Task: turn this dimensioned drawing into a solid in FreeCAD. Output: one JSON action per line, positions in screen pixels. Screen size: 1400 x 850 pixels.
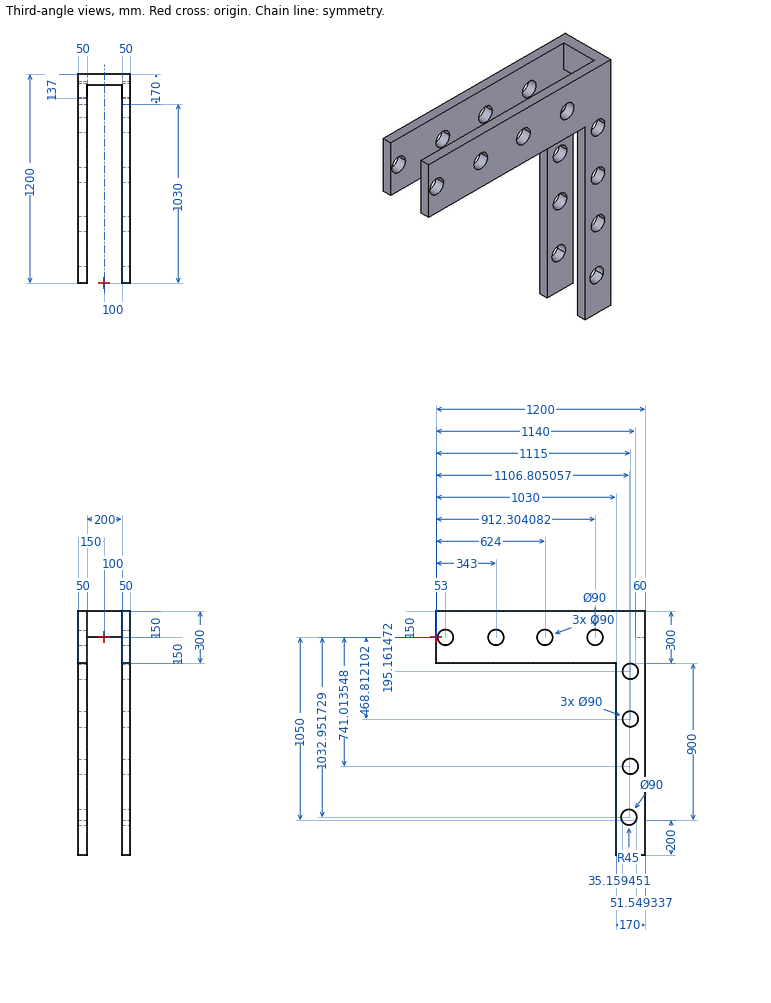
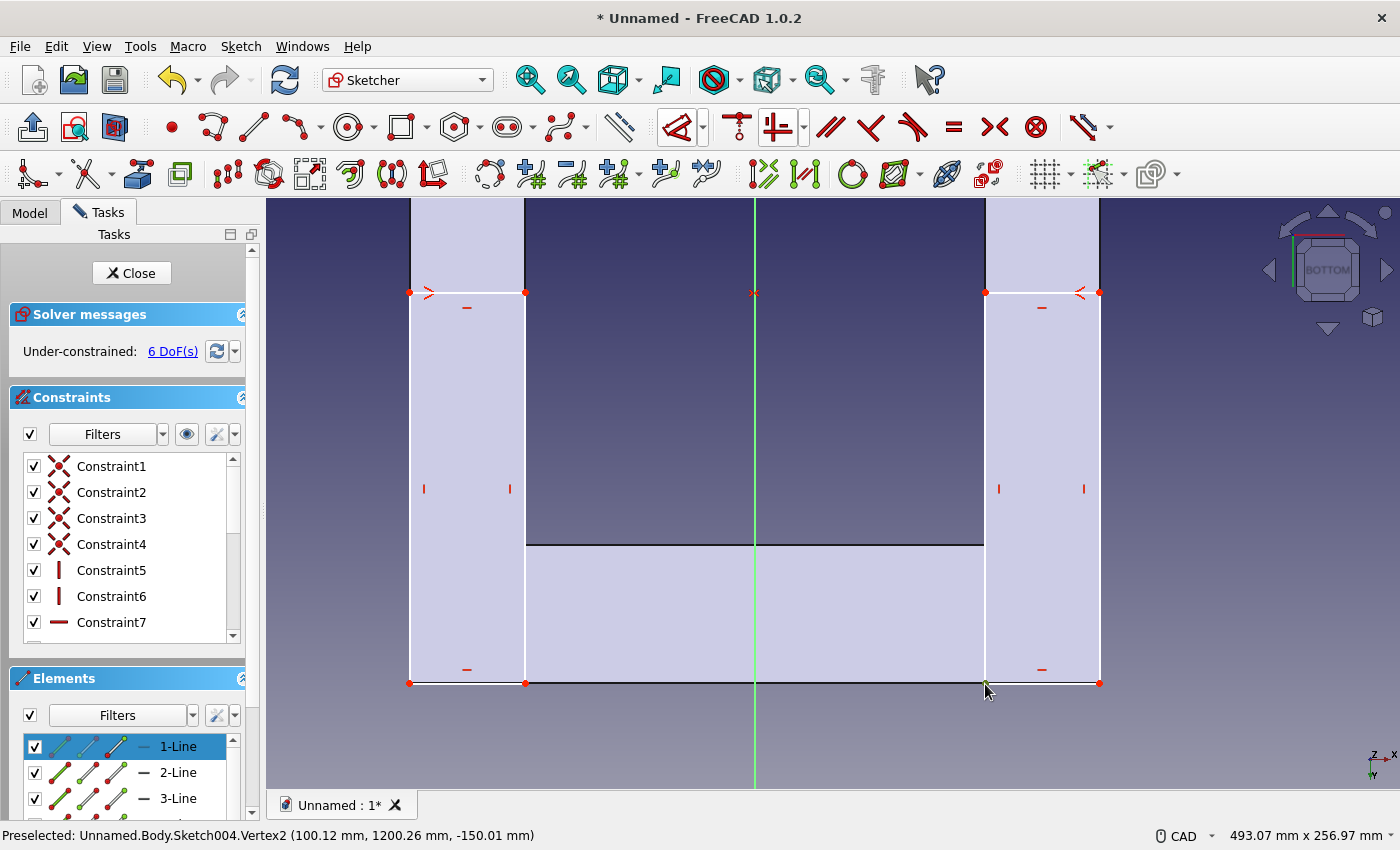
{"action": "left_click", "coordinate": [525, 684]}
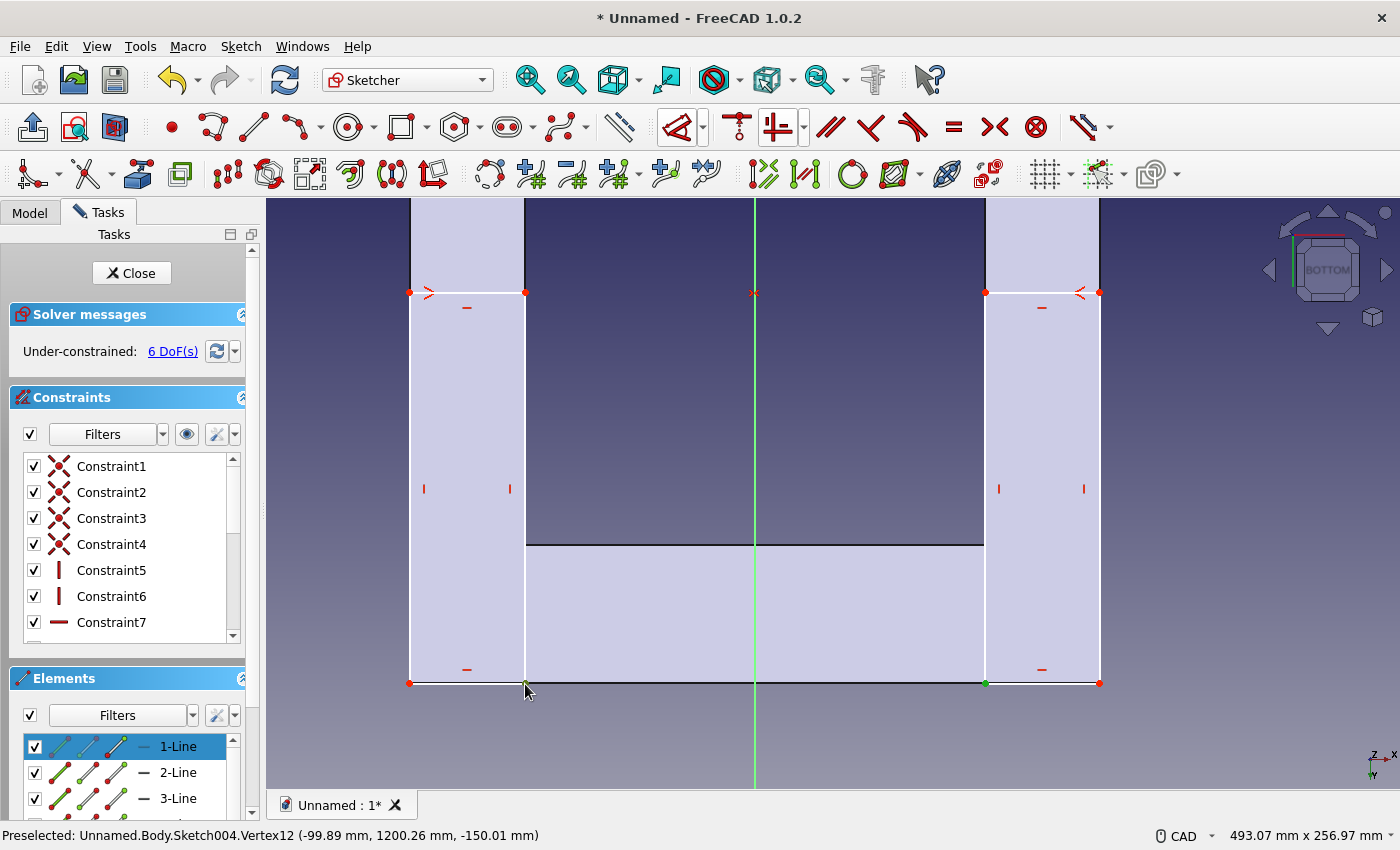
{"action": "left_click", "coordinate": [755, 723]}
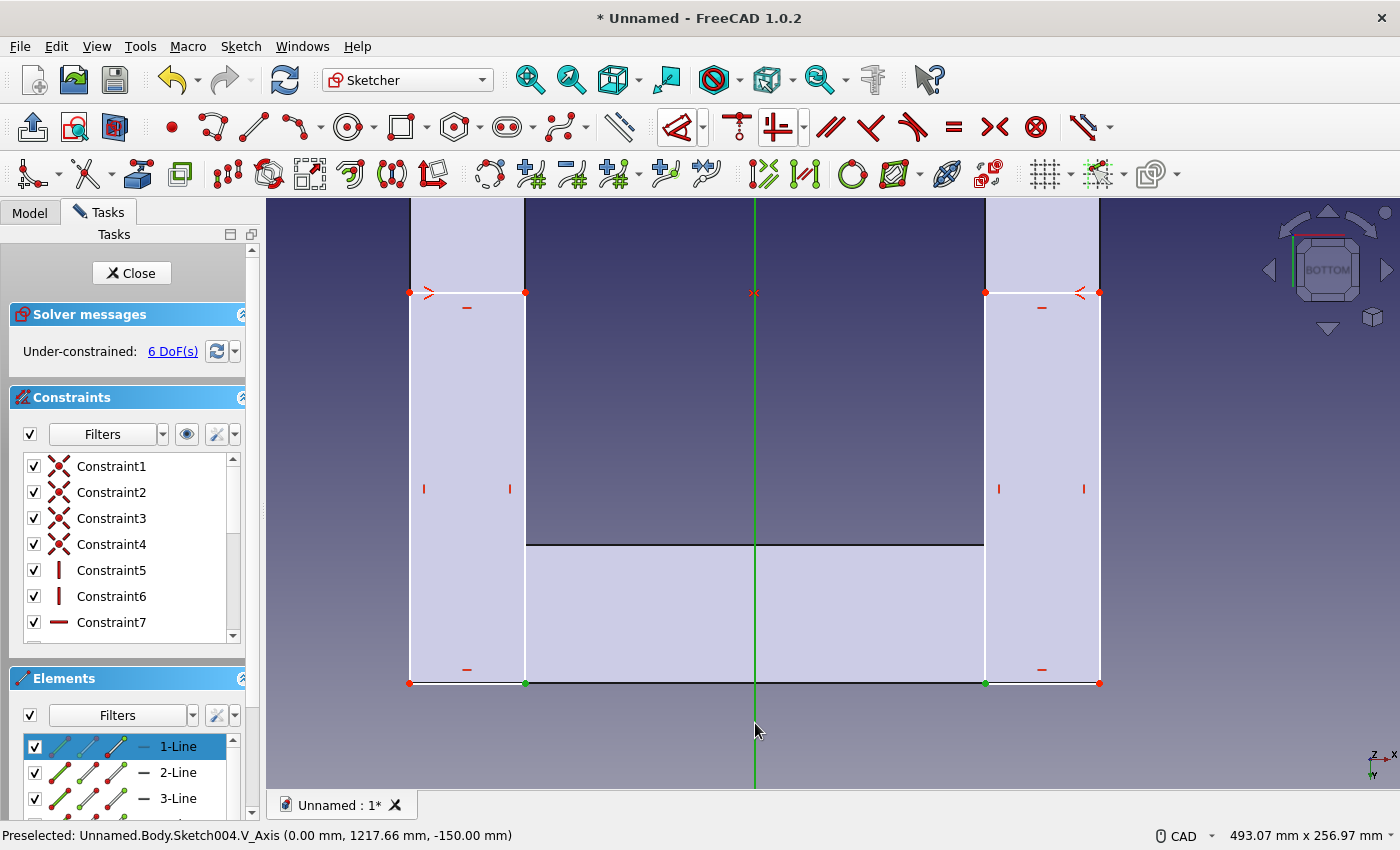
{"action": "left_click", "coordinate": [995, 128]}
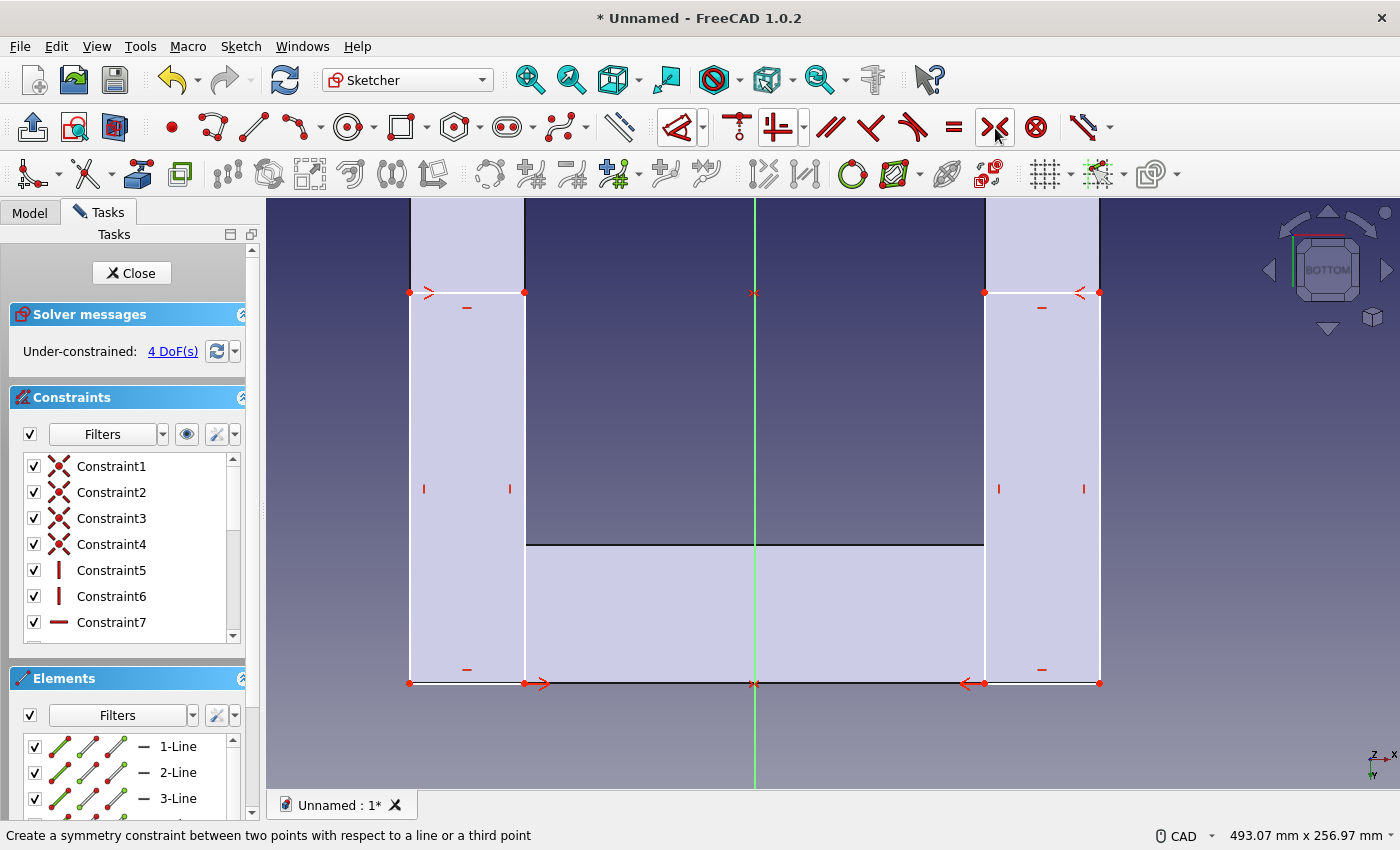
{"action": "left_click", "coordinate": [1019, 684]}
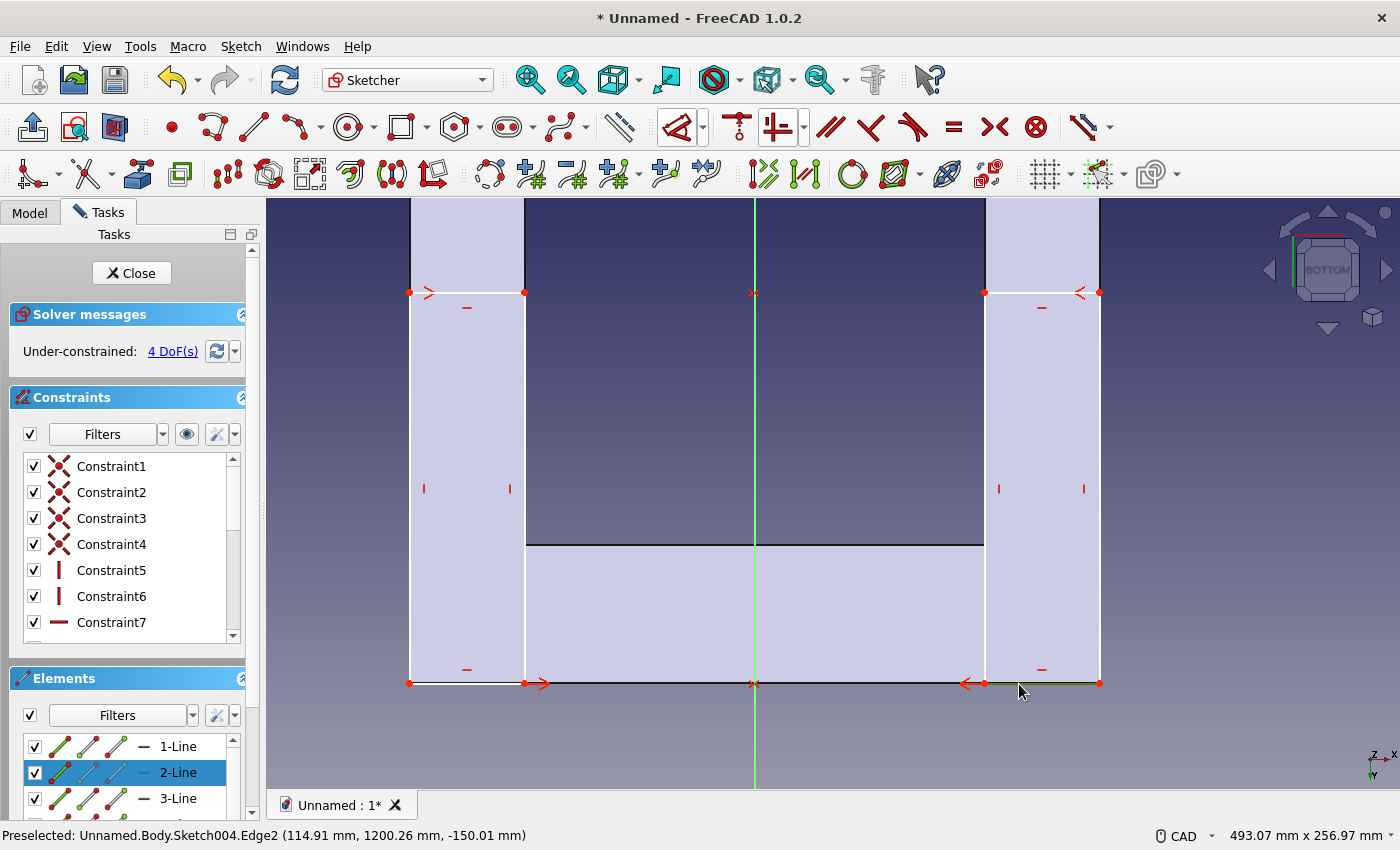
{"action": "left_click", "coordinate": [702, 128]}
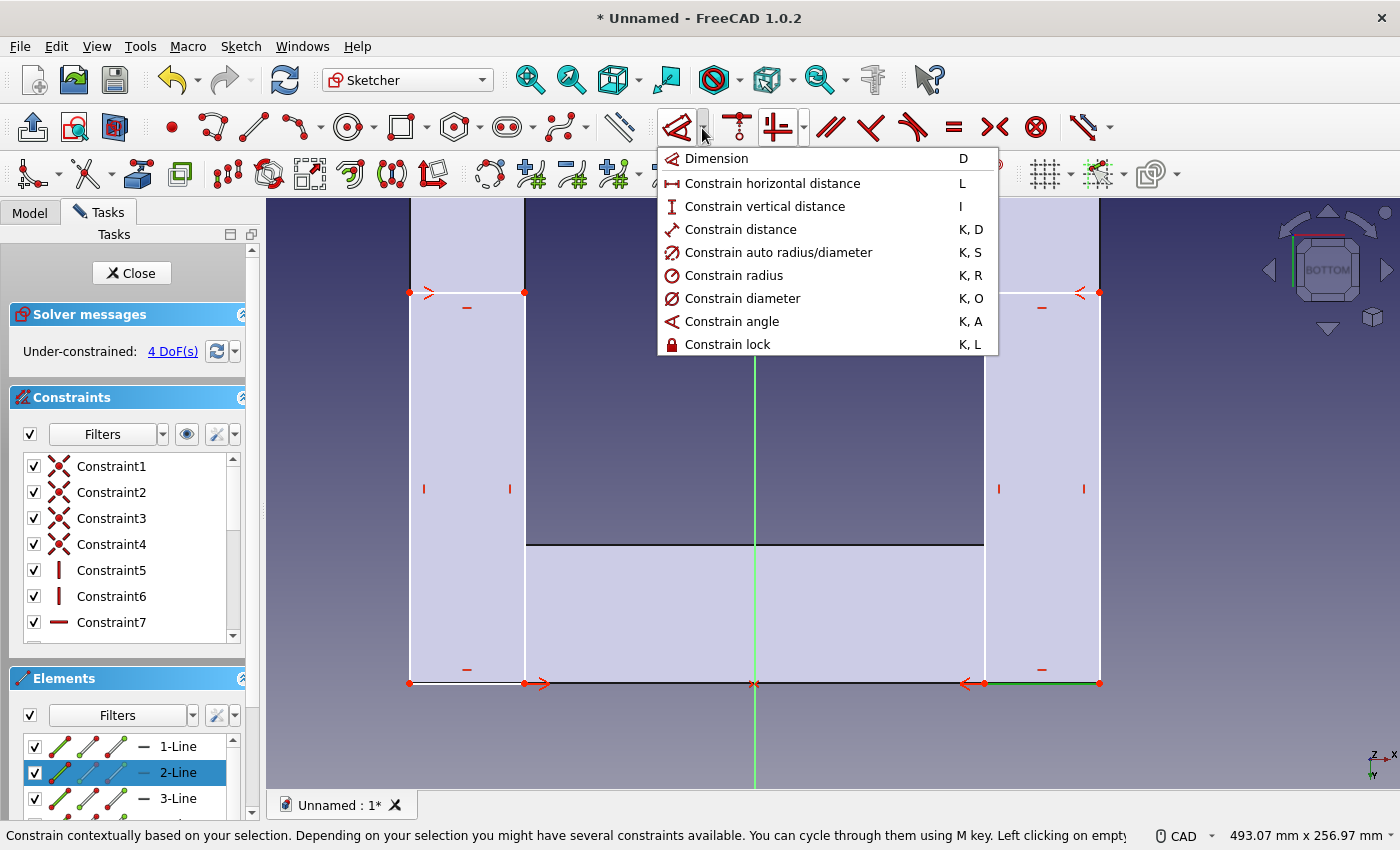
{"action": "left_click", "coordinate": [828, 184]}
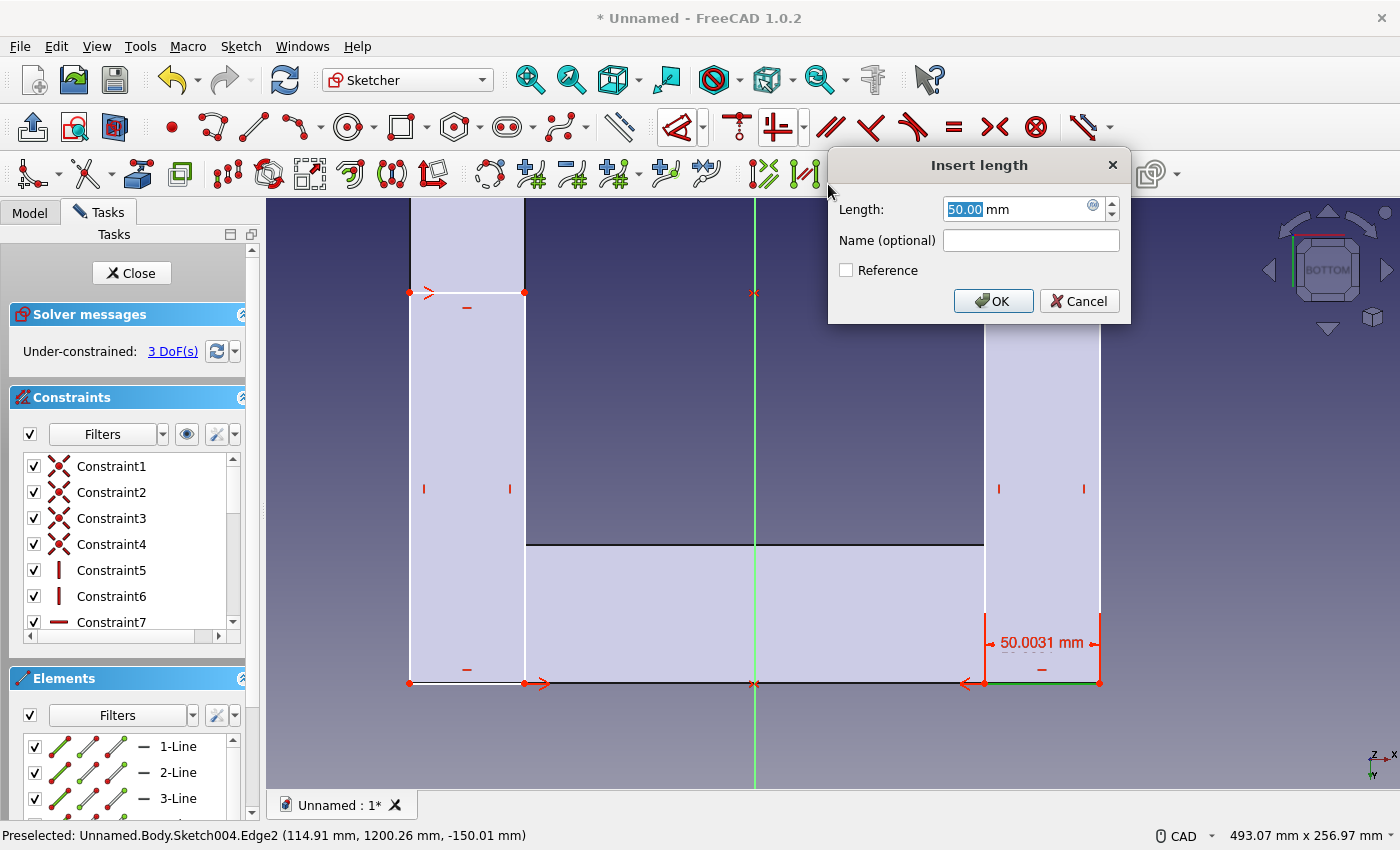
{"action": "type", "text": "50"}
{"action": "key", "text": "Return"}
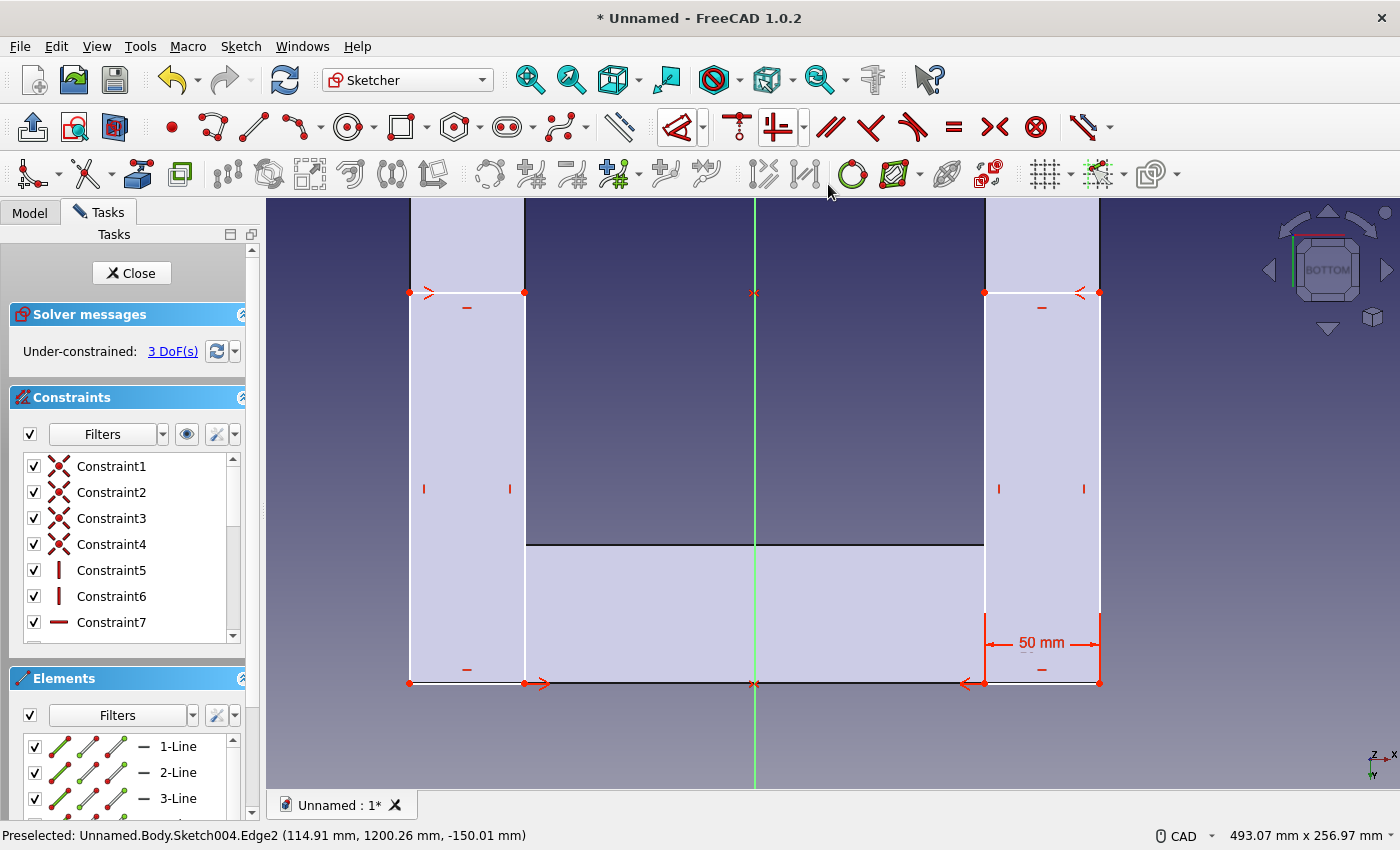
{"action": "left_click", "coordinate": [985, 410]}